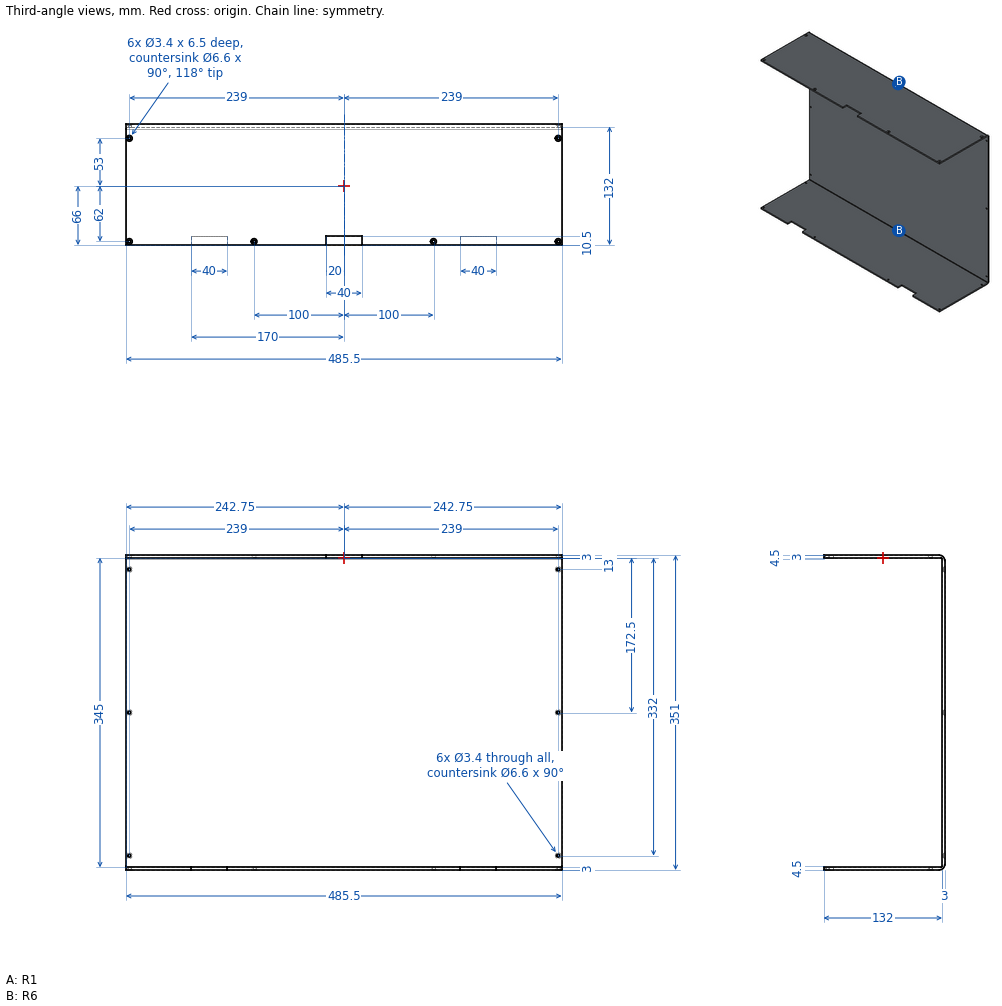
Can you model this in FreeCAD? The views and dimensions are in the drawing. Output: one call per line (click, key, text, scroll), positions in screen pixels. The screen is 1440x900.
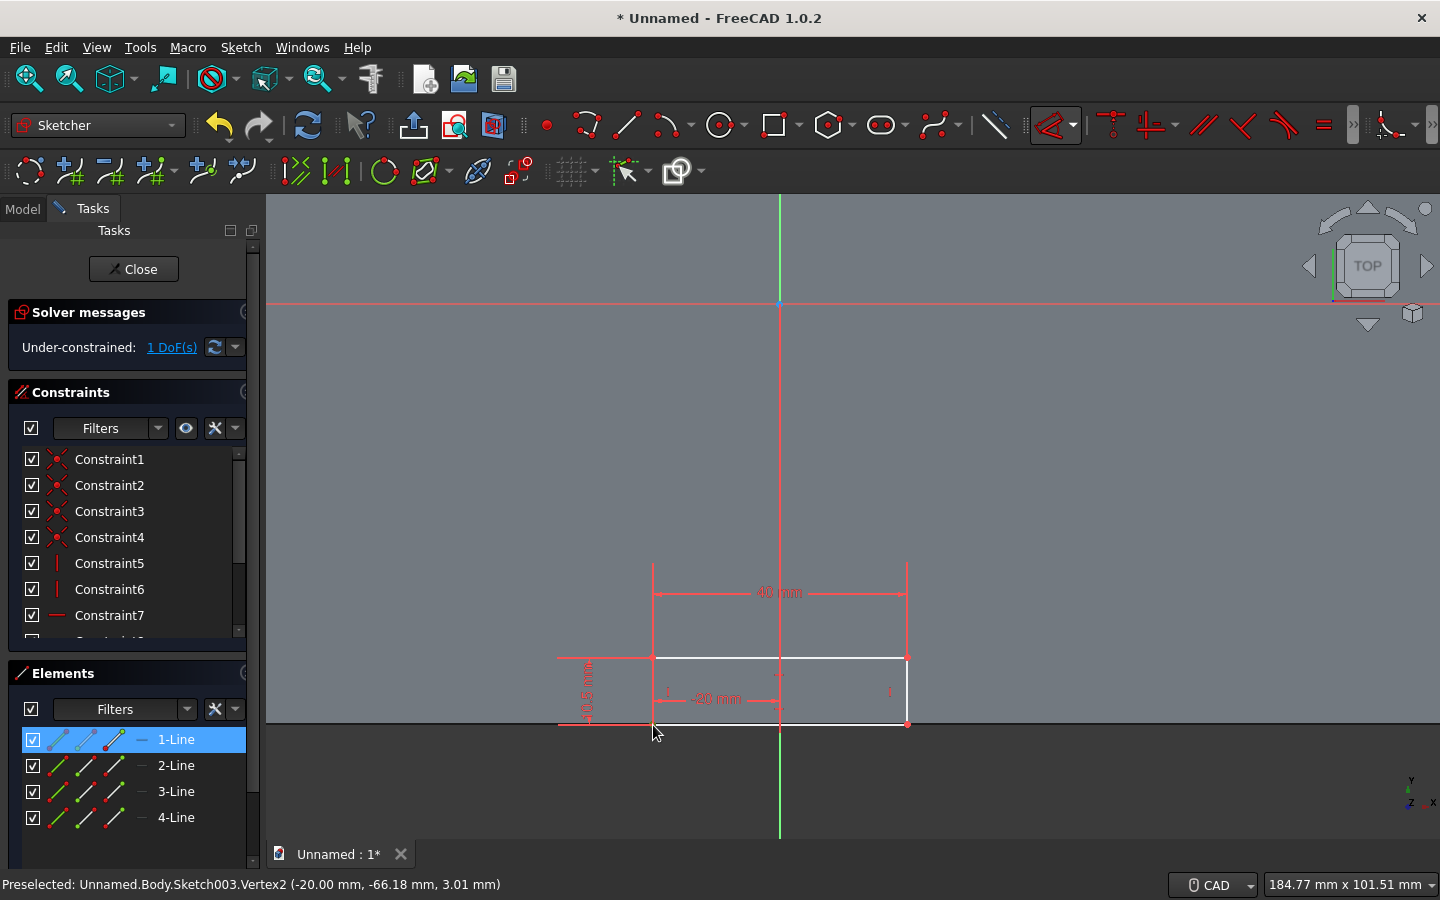
click(1076, 126)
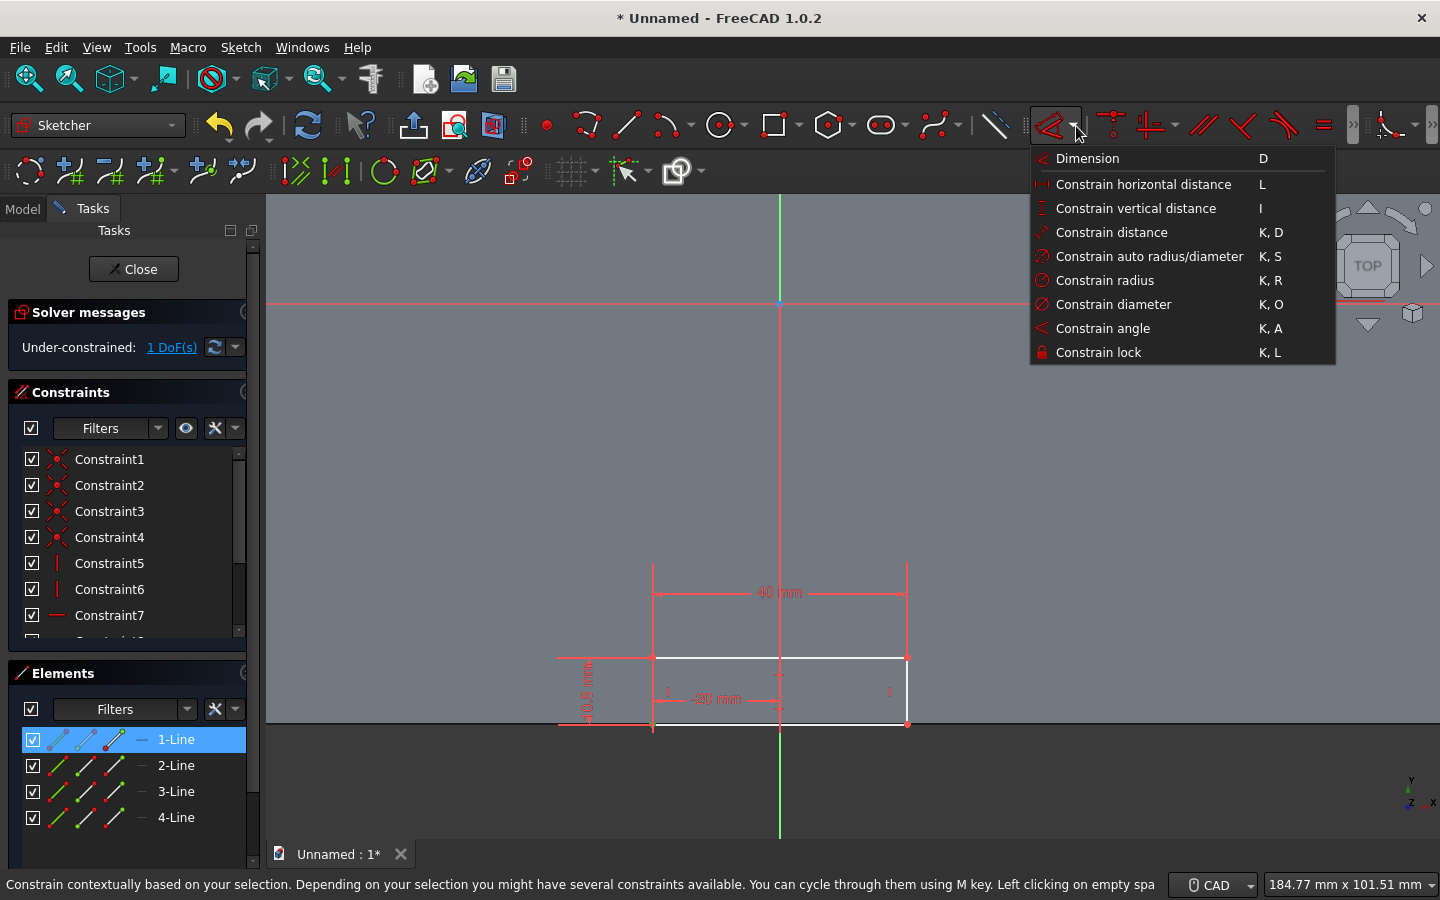
click(1183, 208)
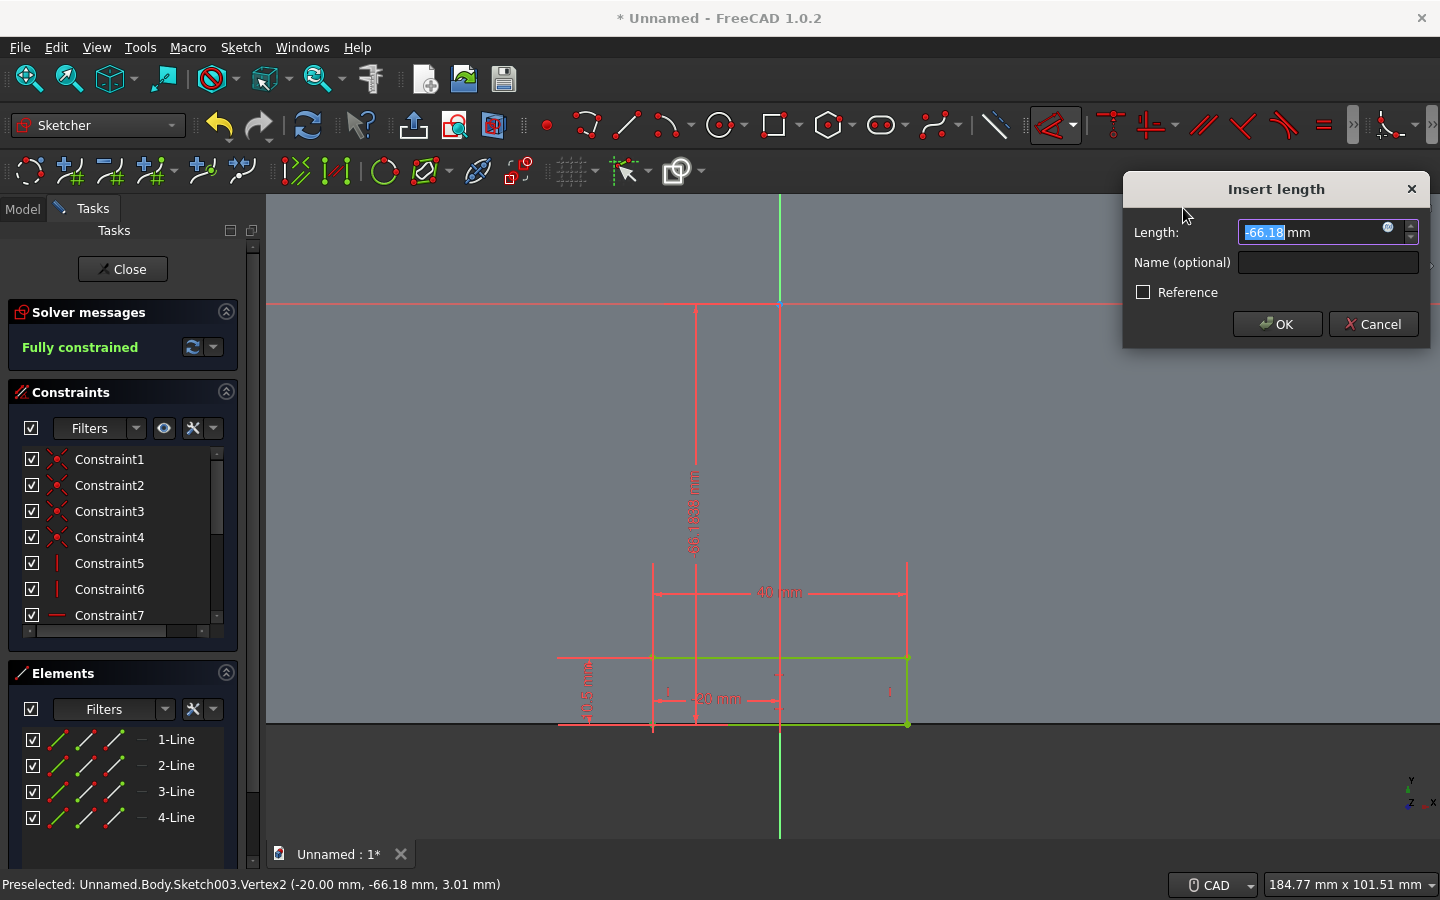
text(-66)
key(Return)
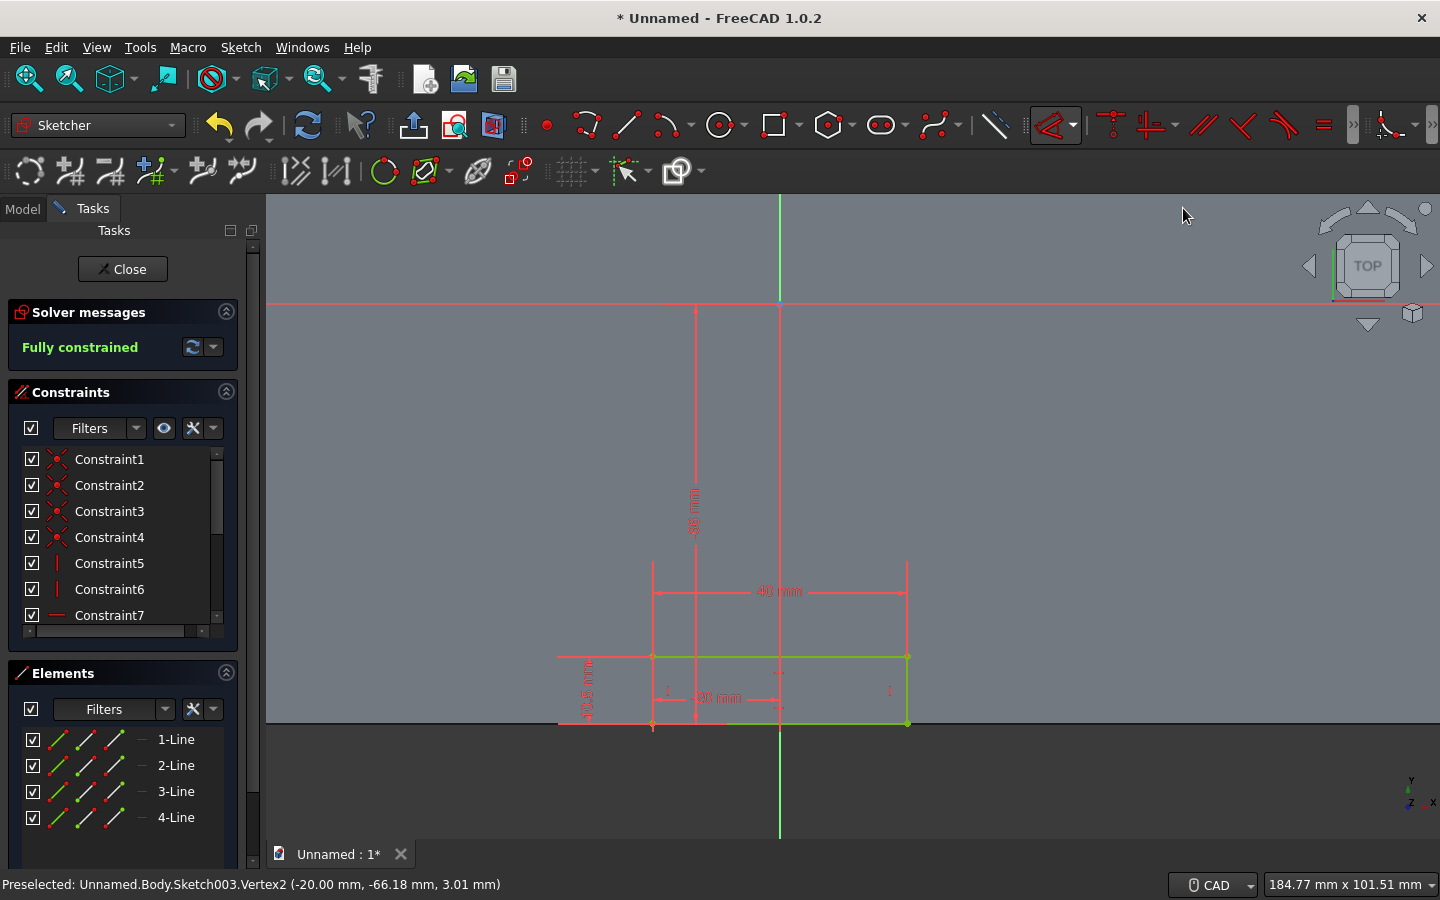
click(123, 269)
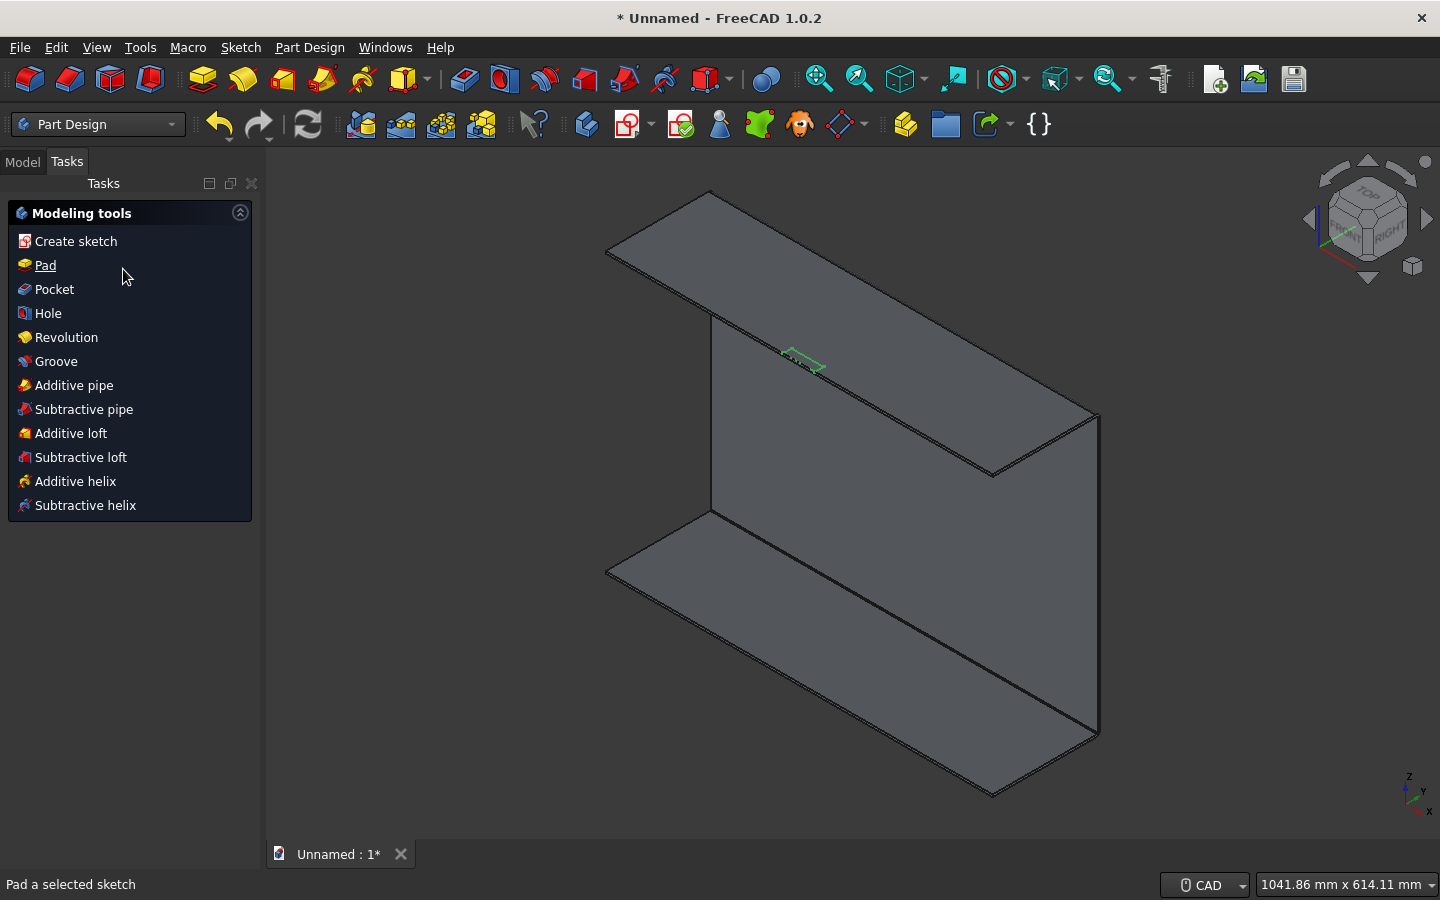
click(466, 80)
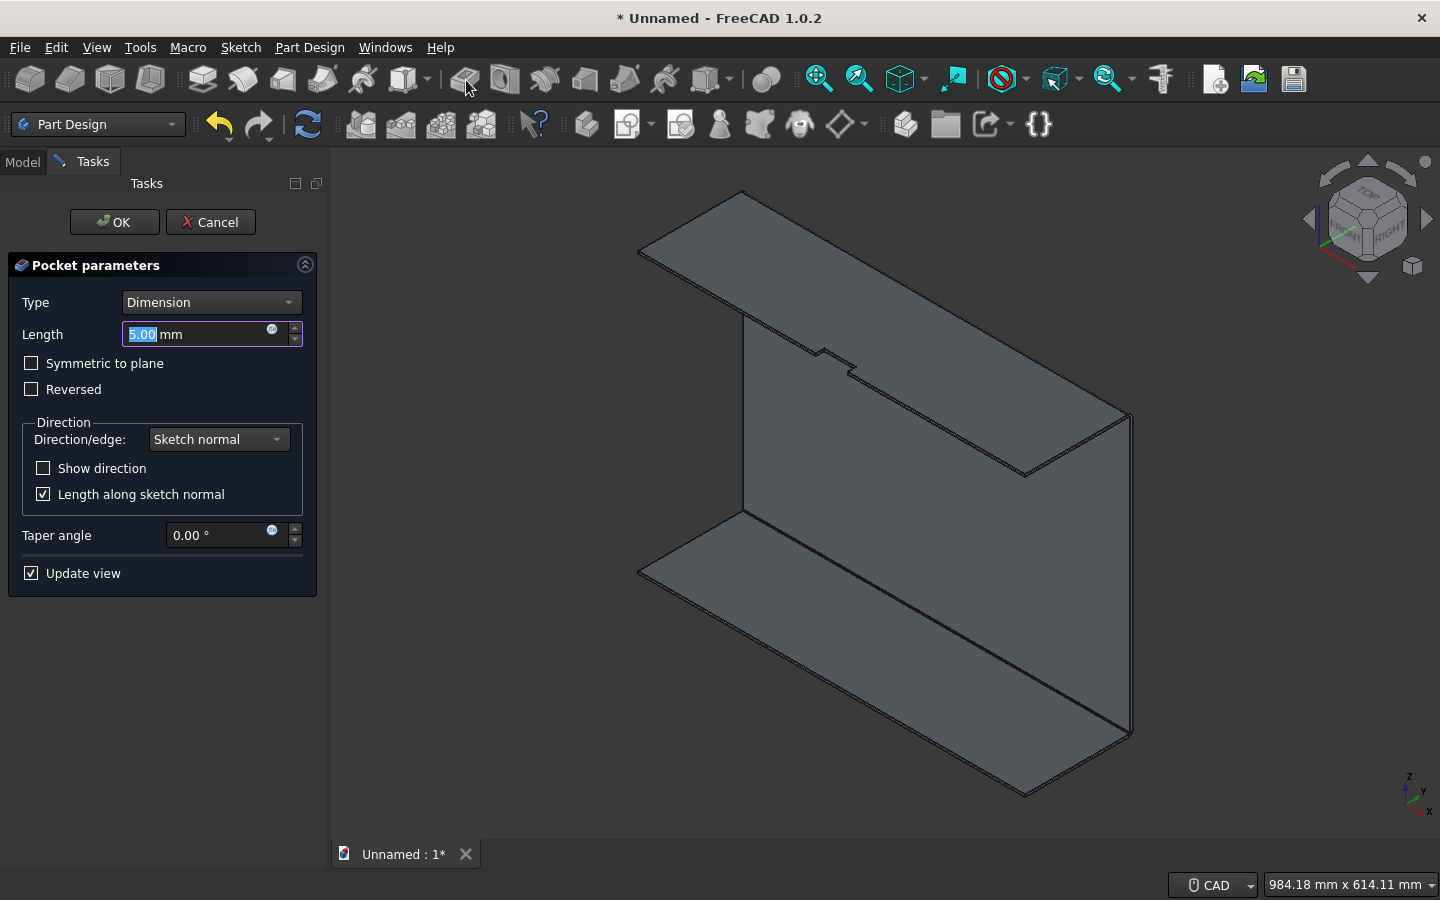
text(4.5)
key(Tab)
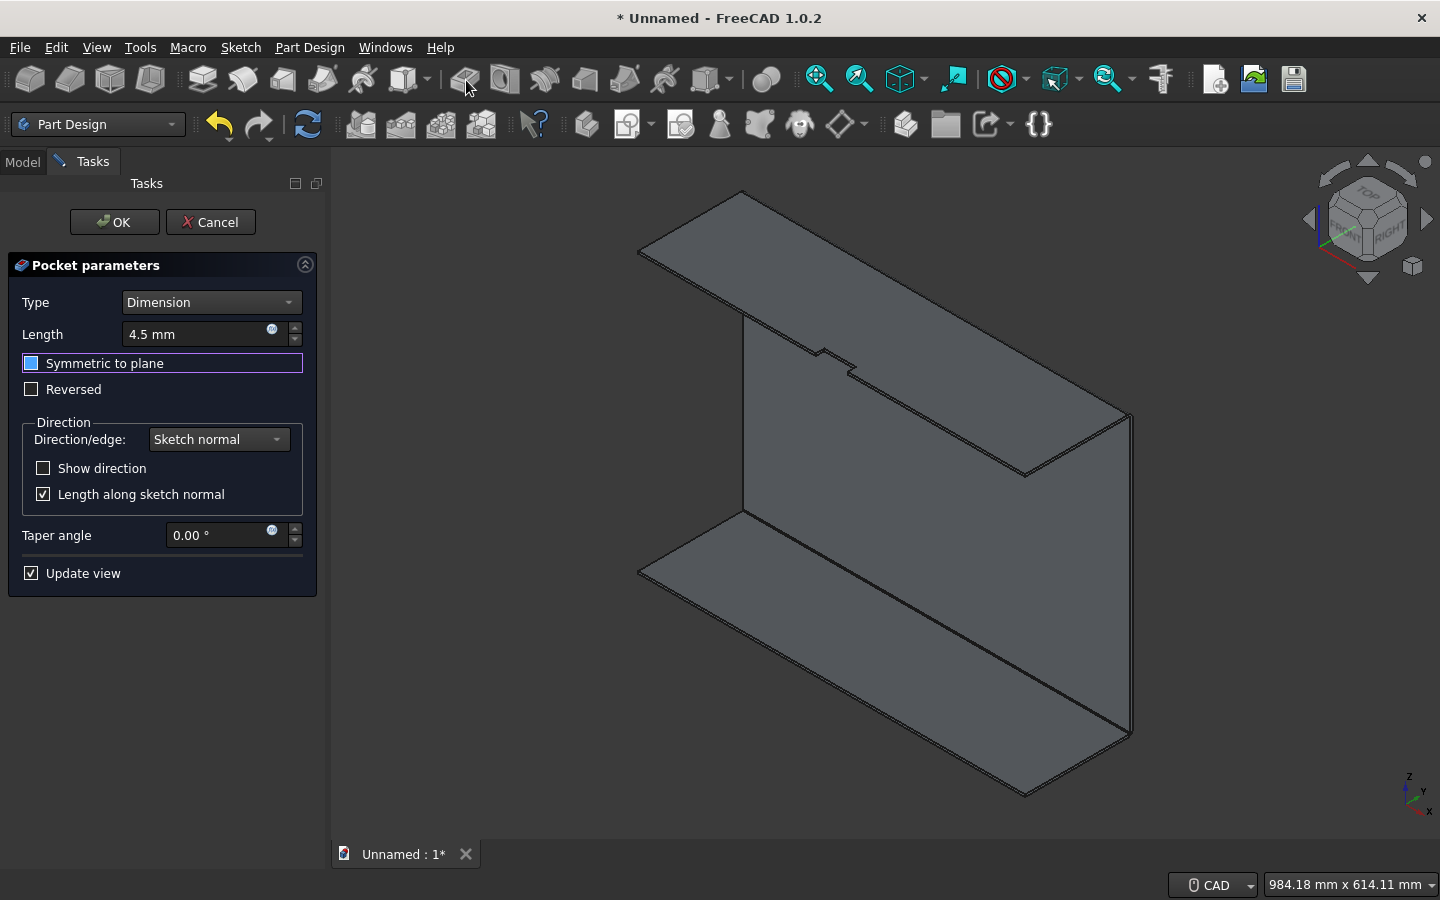
click(115, 222)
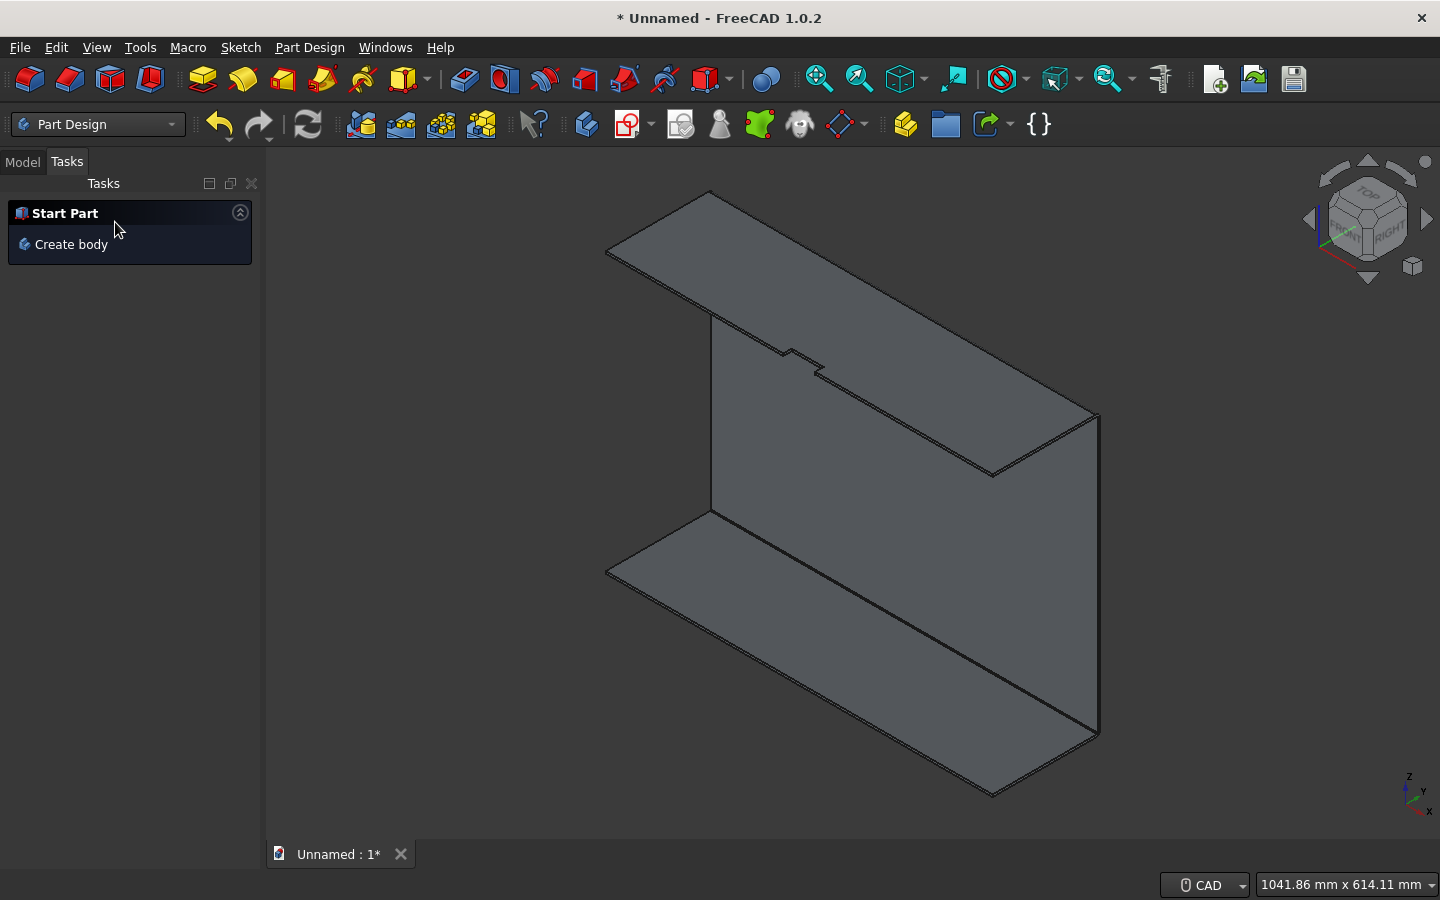
key(5)